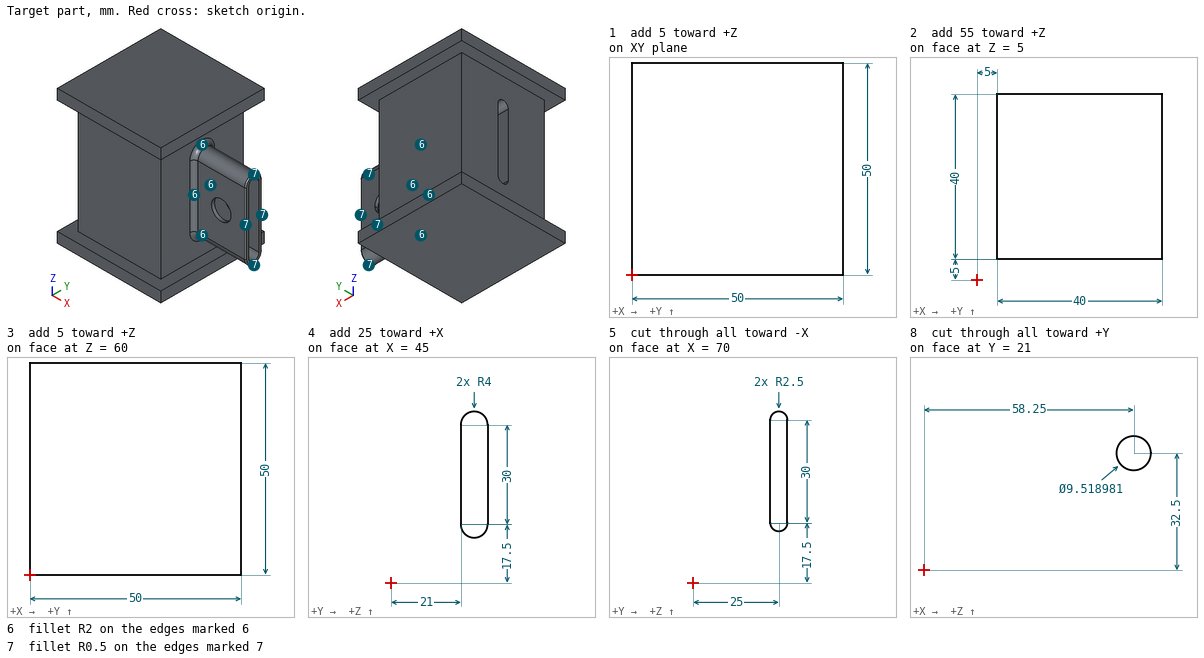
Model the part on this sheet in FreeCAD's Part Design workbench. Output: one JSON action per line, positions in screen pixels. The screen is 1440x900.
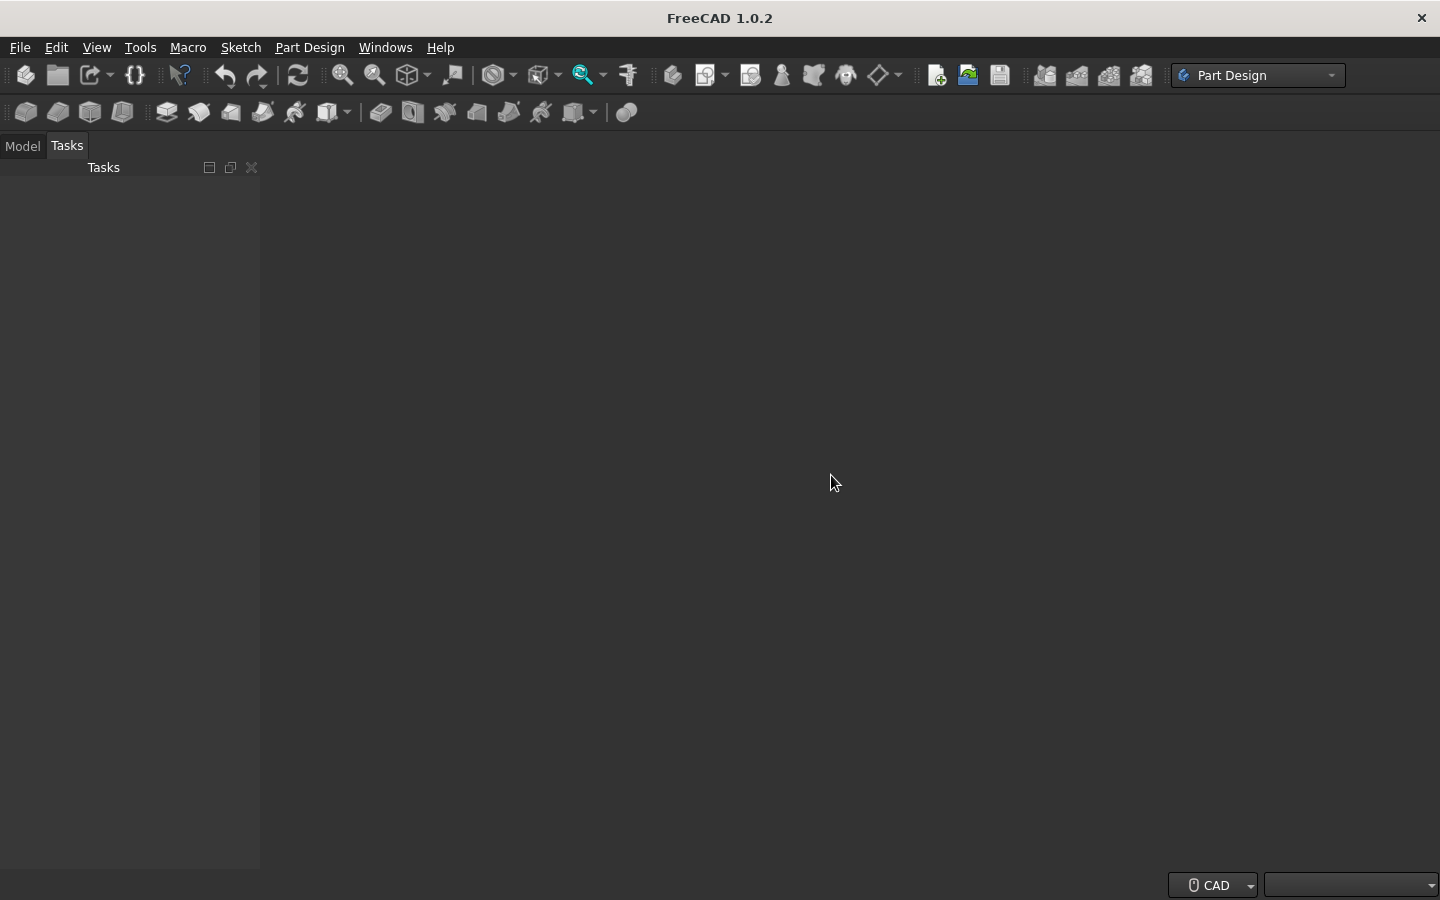
{"action": "left_click", "coordinate": [936, 76]}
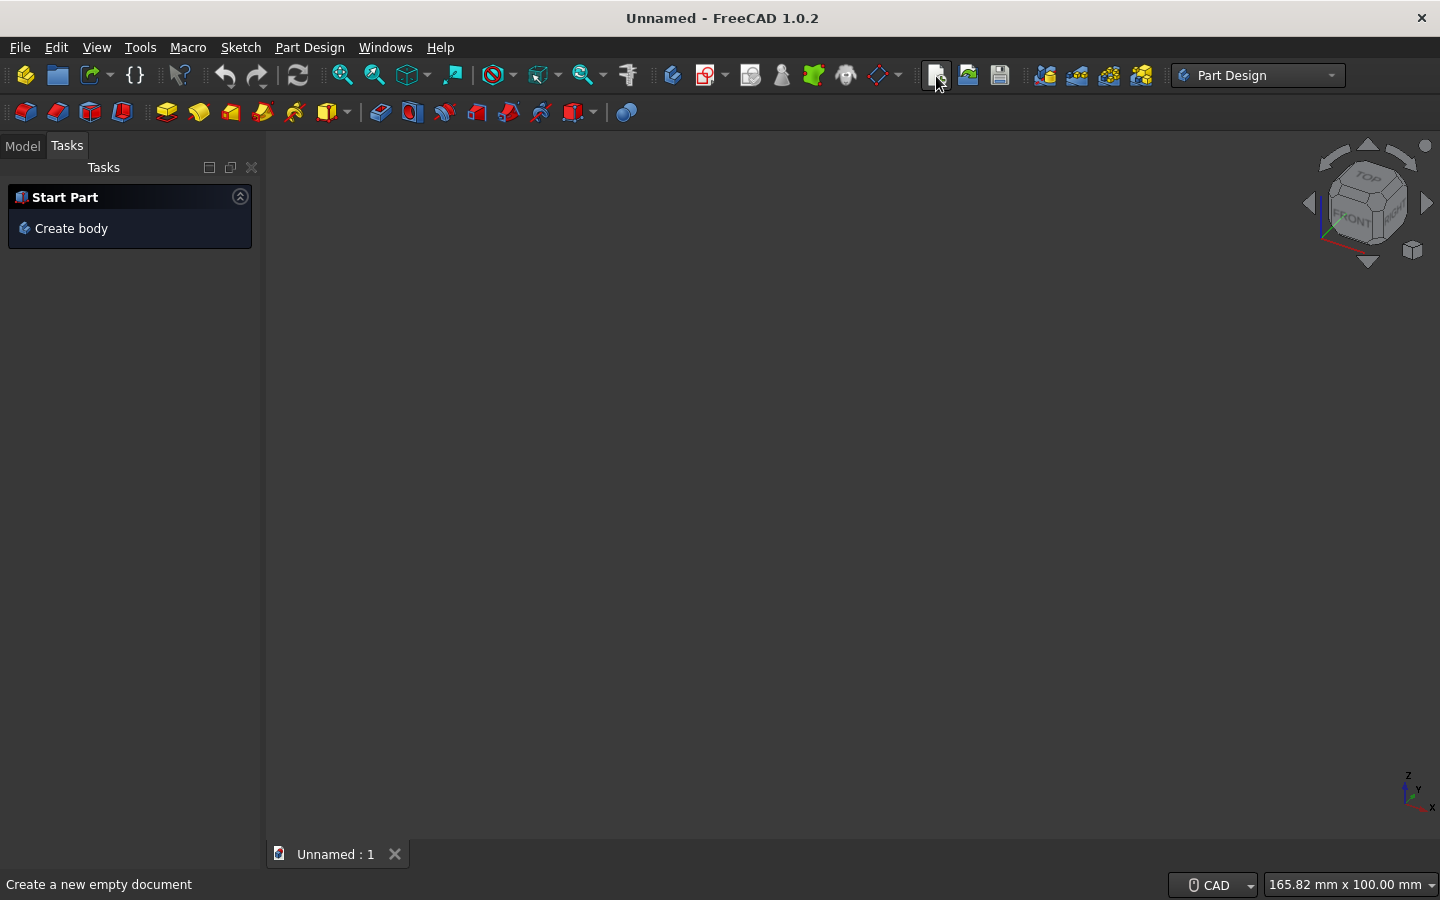
{"action": "left_click", "coordinate": [706, 76]}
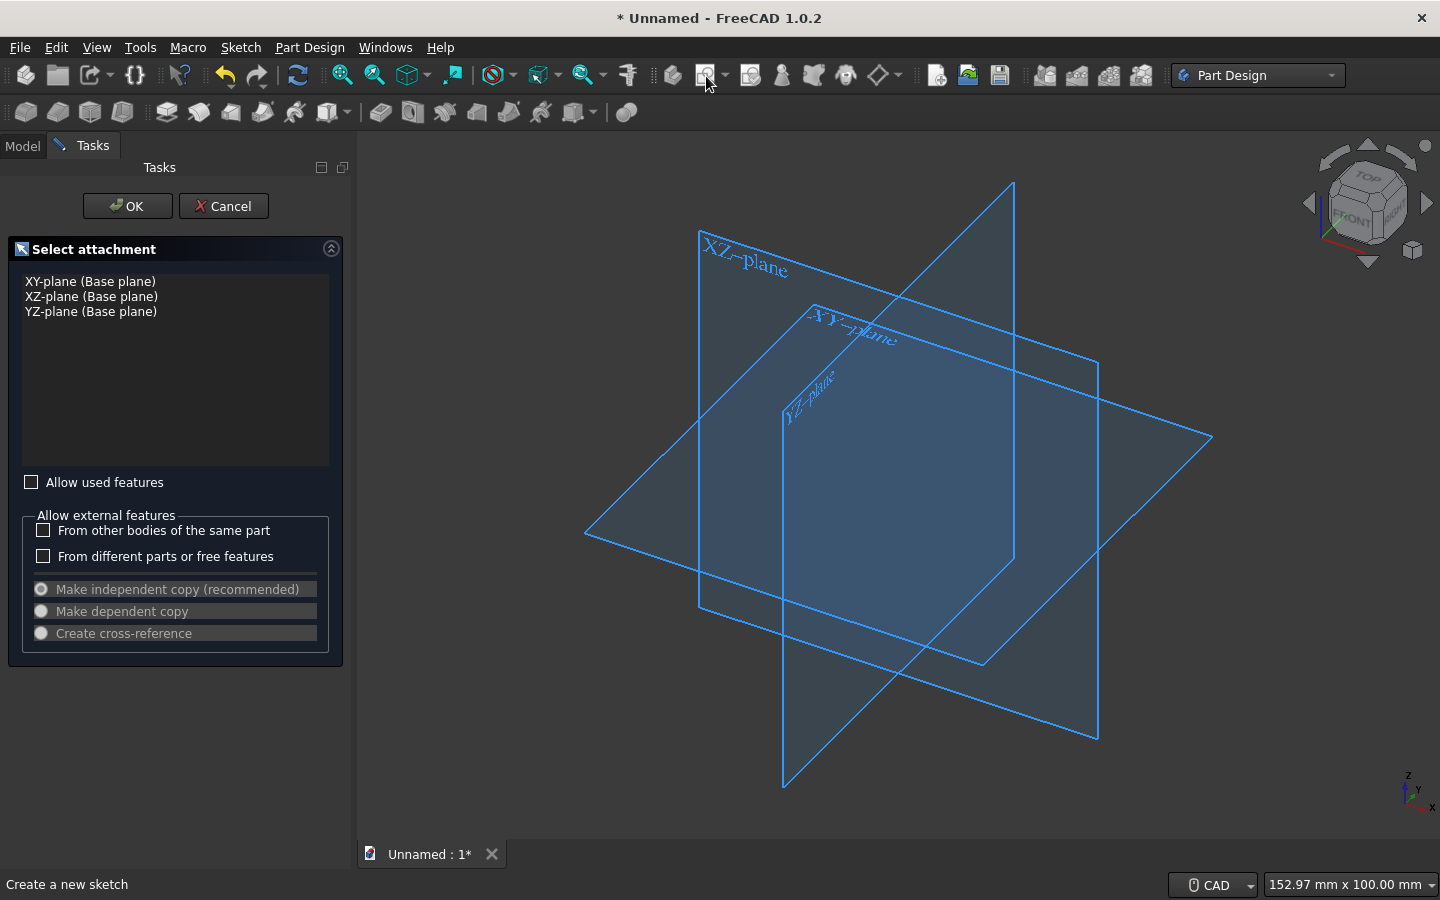
{"action": "left_click", "coordinate": [82, 282]}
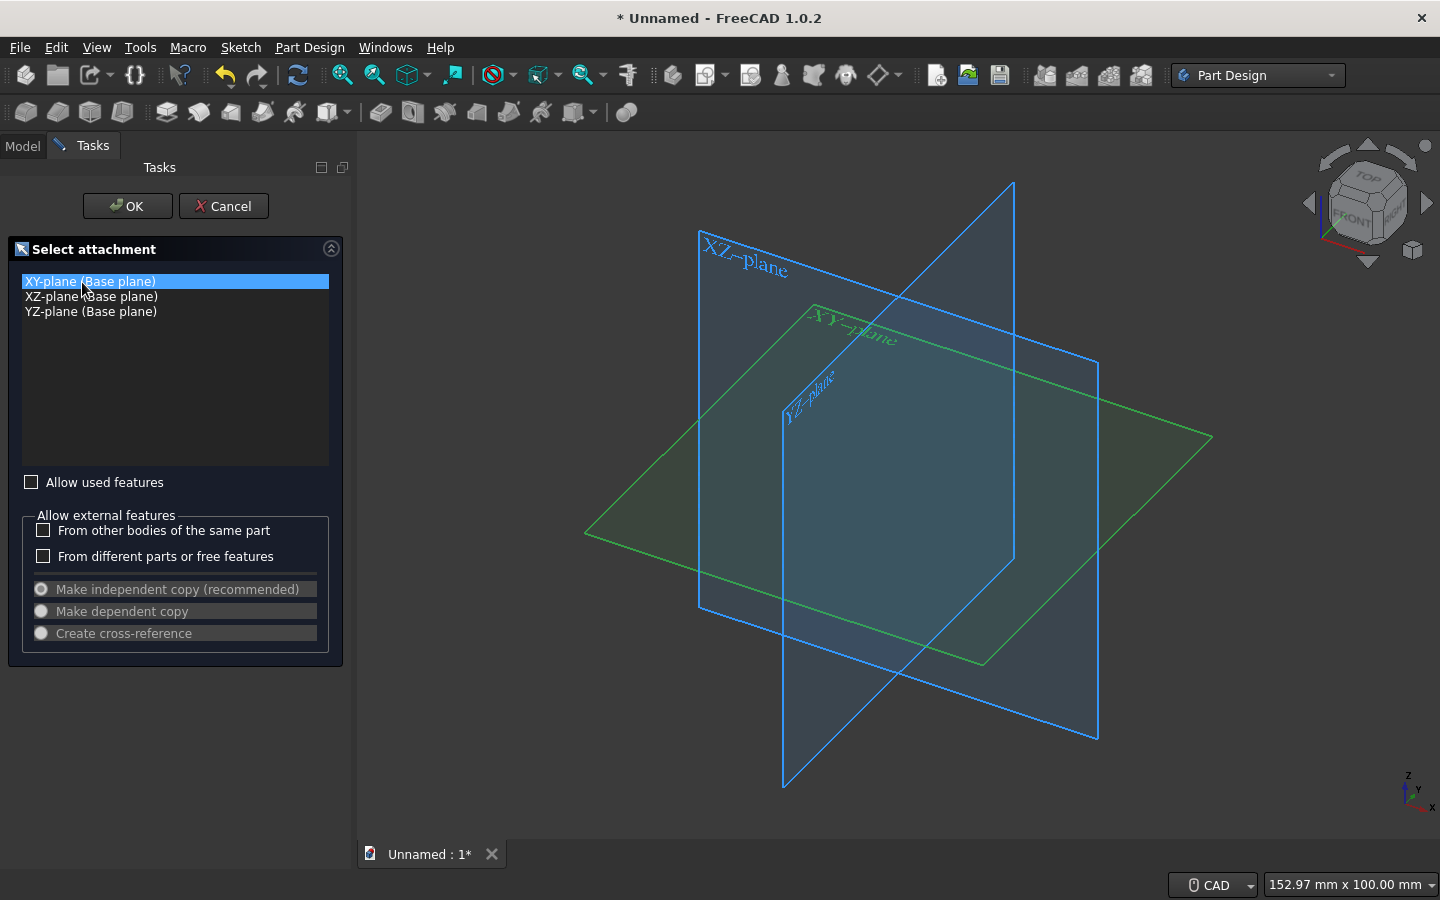
{"action": "left_click", "coordinate": [128, 206]}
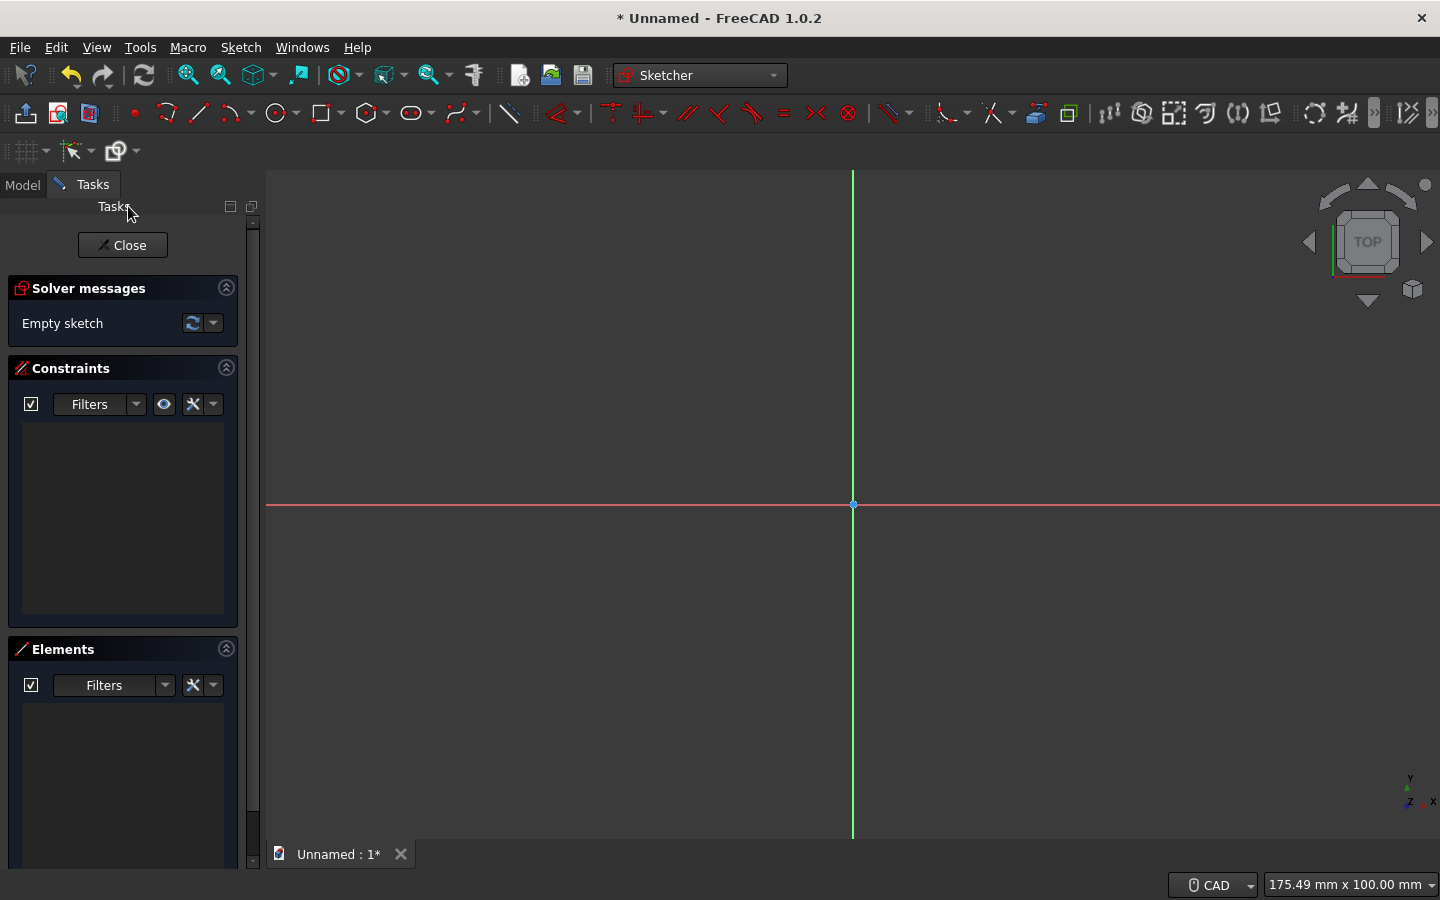
{"action": "scroll", "coordinate": [294, 811], "scroll_direction": "down", "scroll_amount": 1}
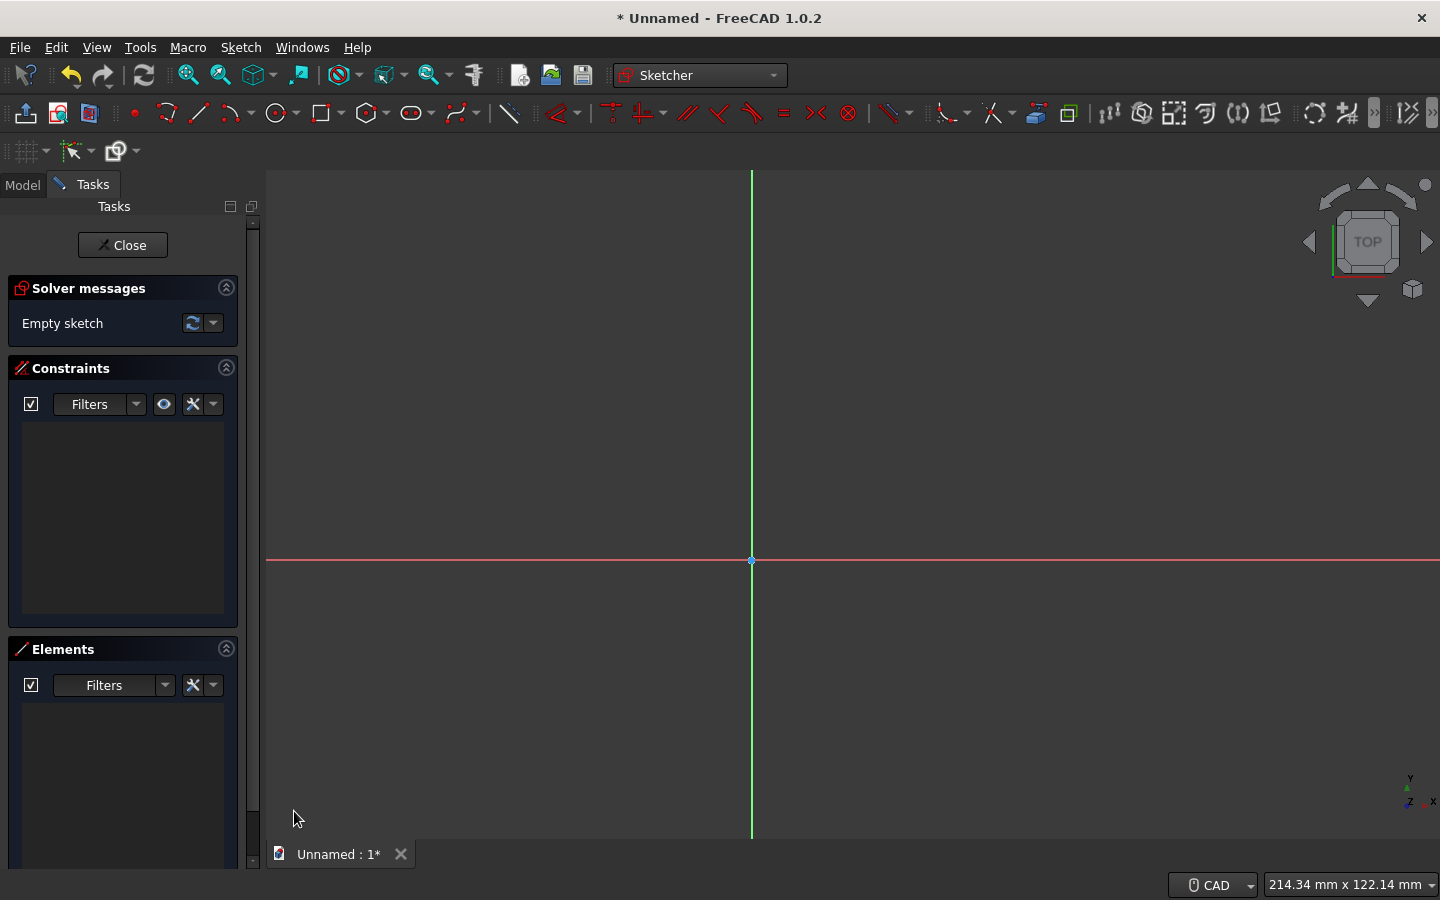
{"action": "scroll", "coordinate": [1100, 258], "scroll_direction": "up", "scroll_amount": 2}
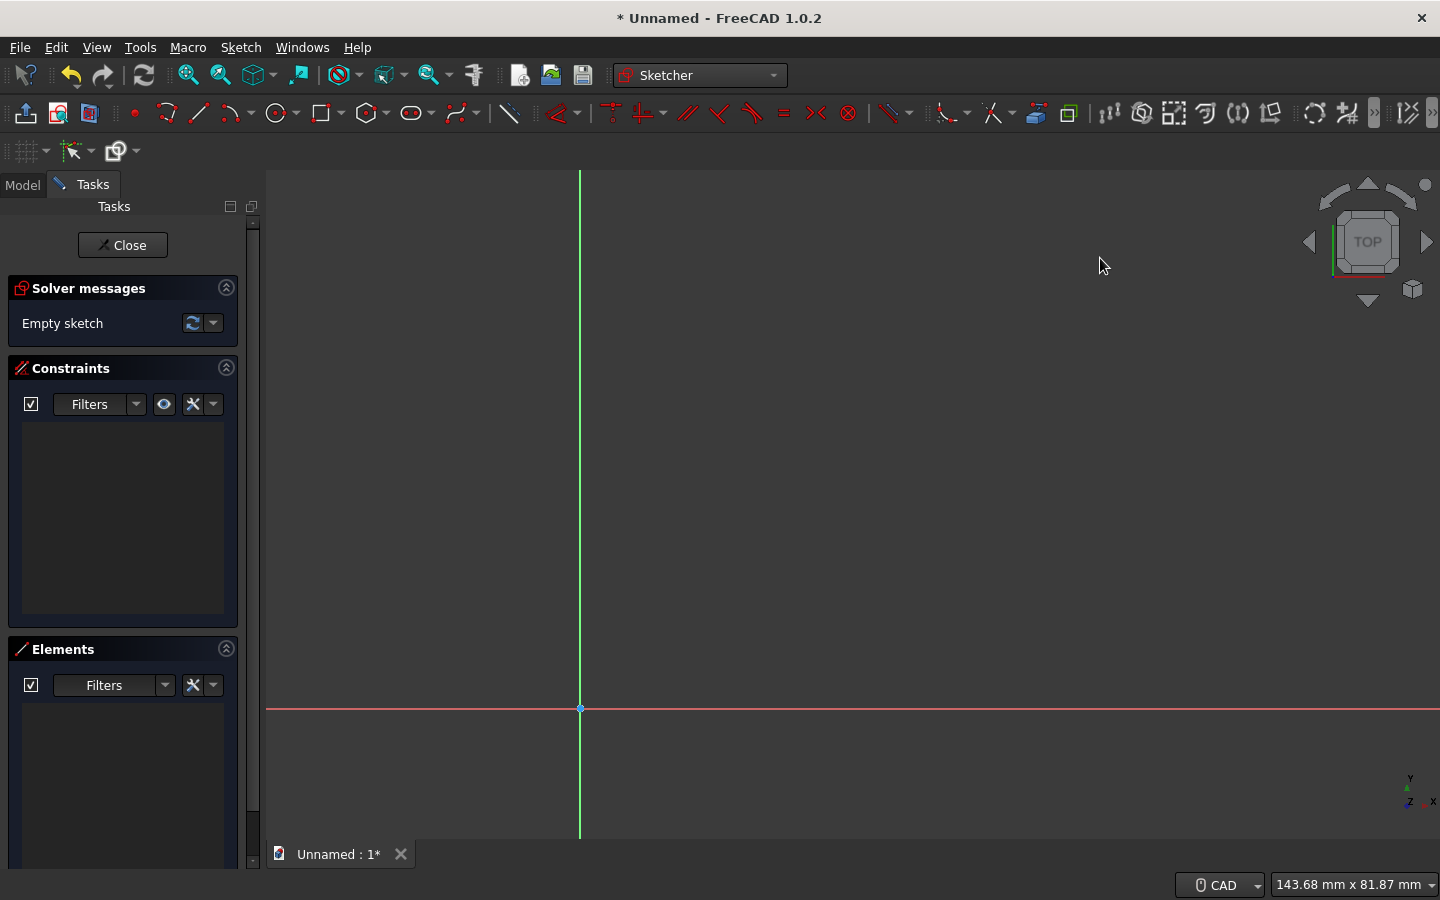
{"action": "left_click", "coordinate": [322, 114]}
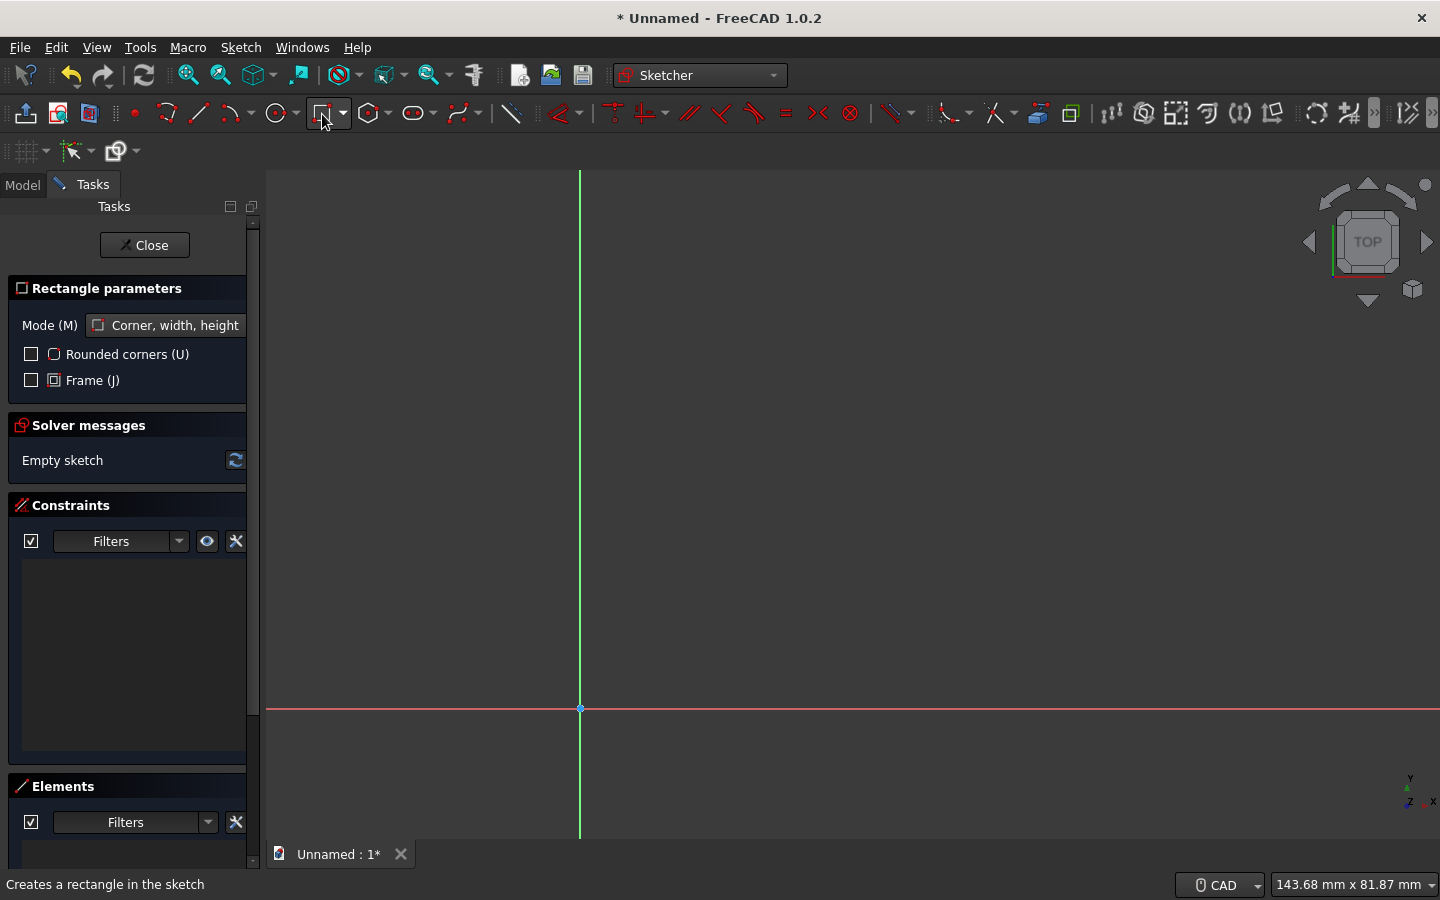
{"action": "left_click", "coordinate": [580, 709]}
{"action": "left_click", "coordinate": [989, 300]}
{"action": "key", "text": "Escape"}